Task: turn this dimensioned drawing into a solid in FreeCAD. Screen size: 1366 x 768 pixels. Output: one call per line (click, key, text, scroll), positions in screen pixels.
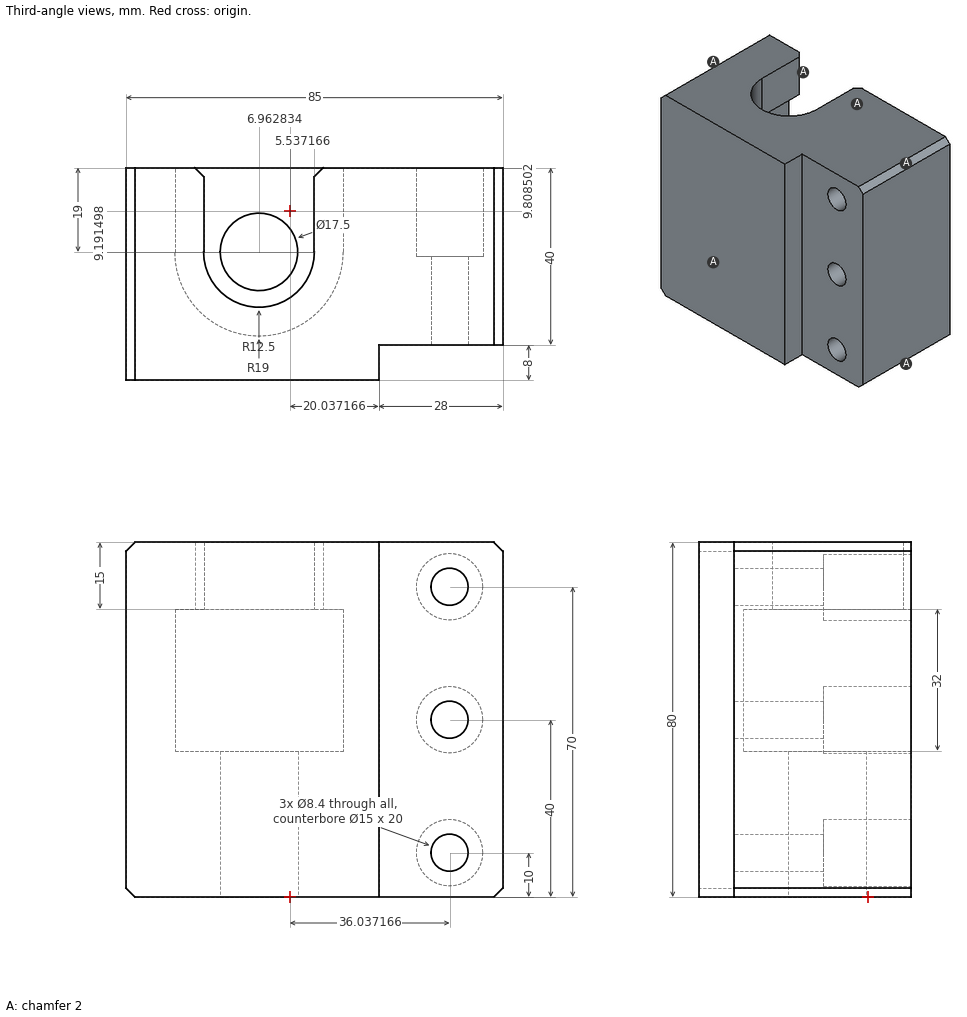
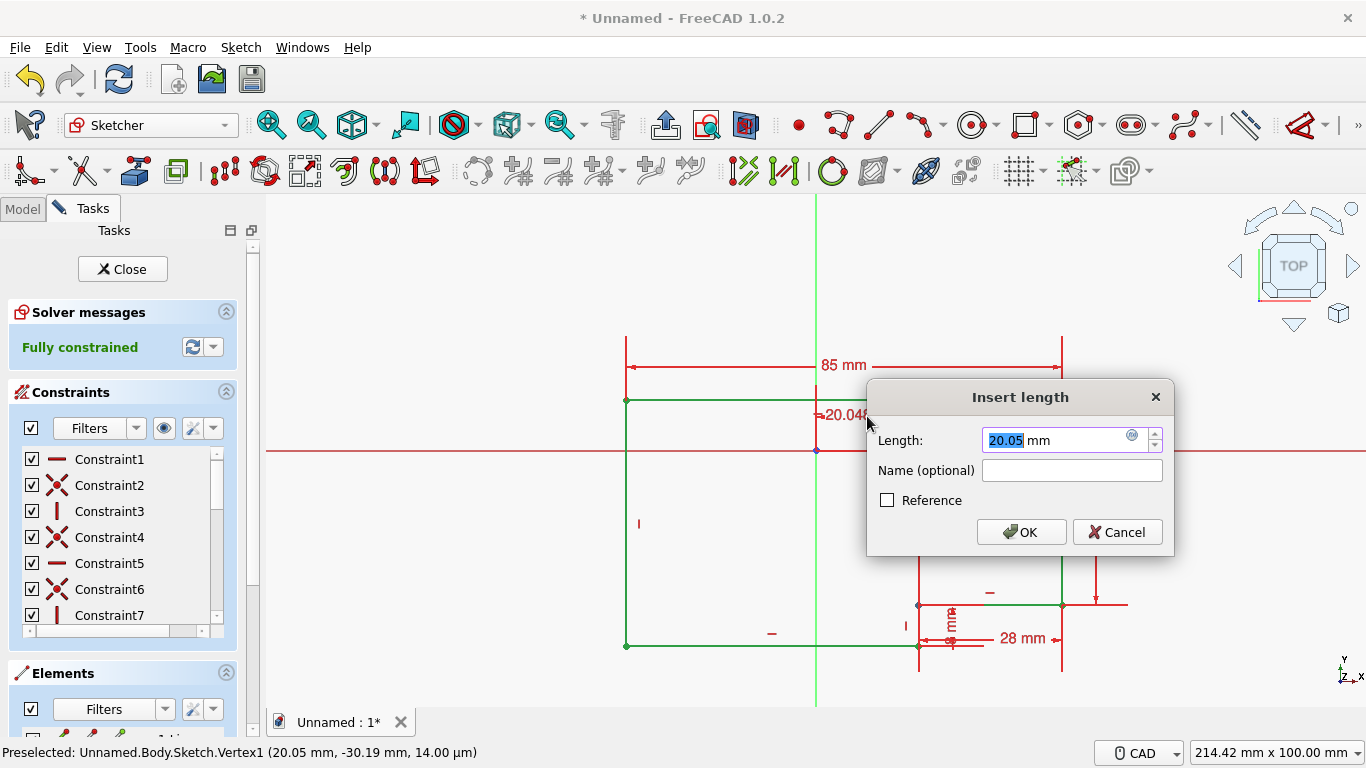
text(20.037166)
key(Return)
key(Escape)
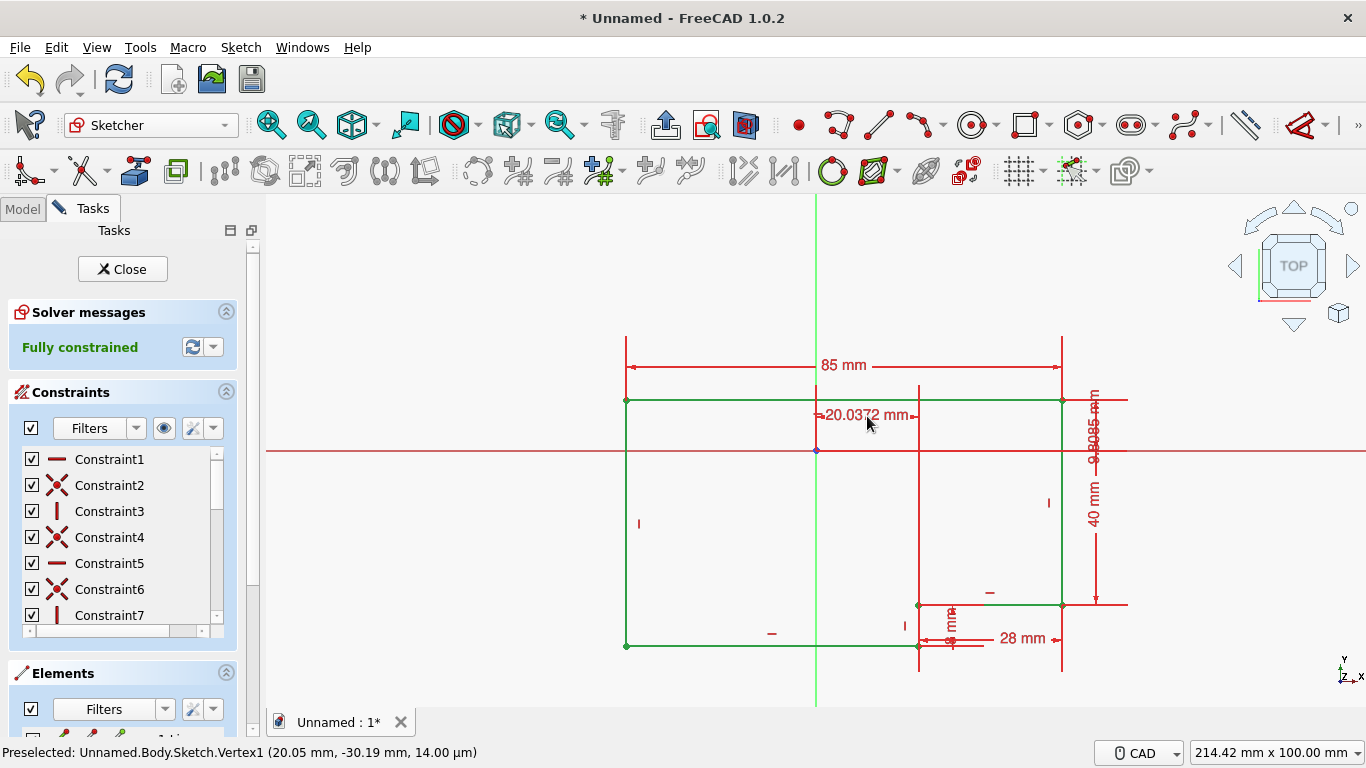
click(123, 269)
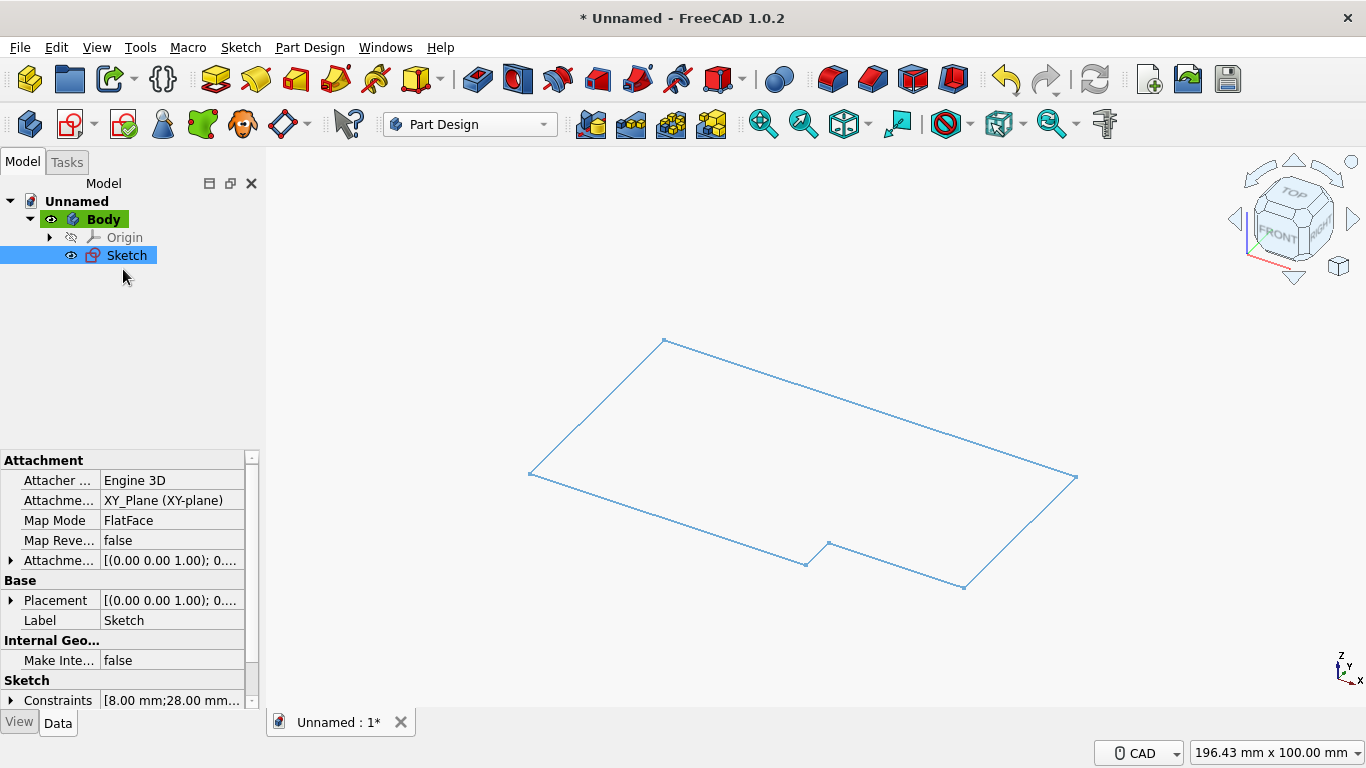
click(216, 80)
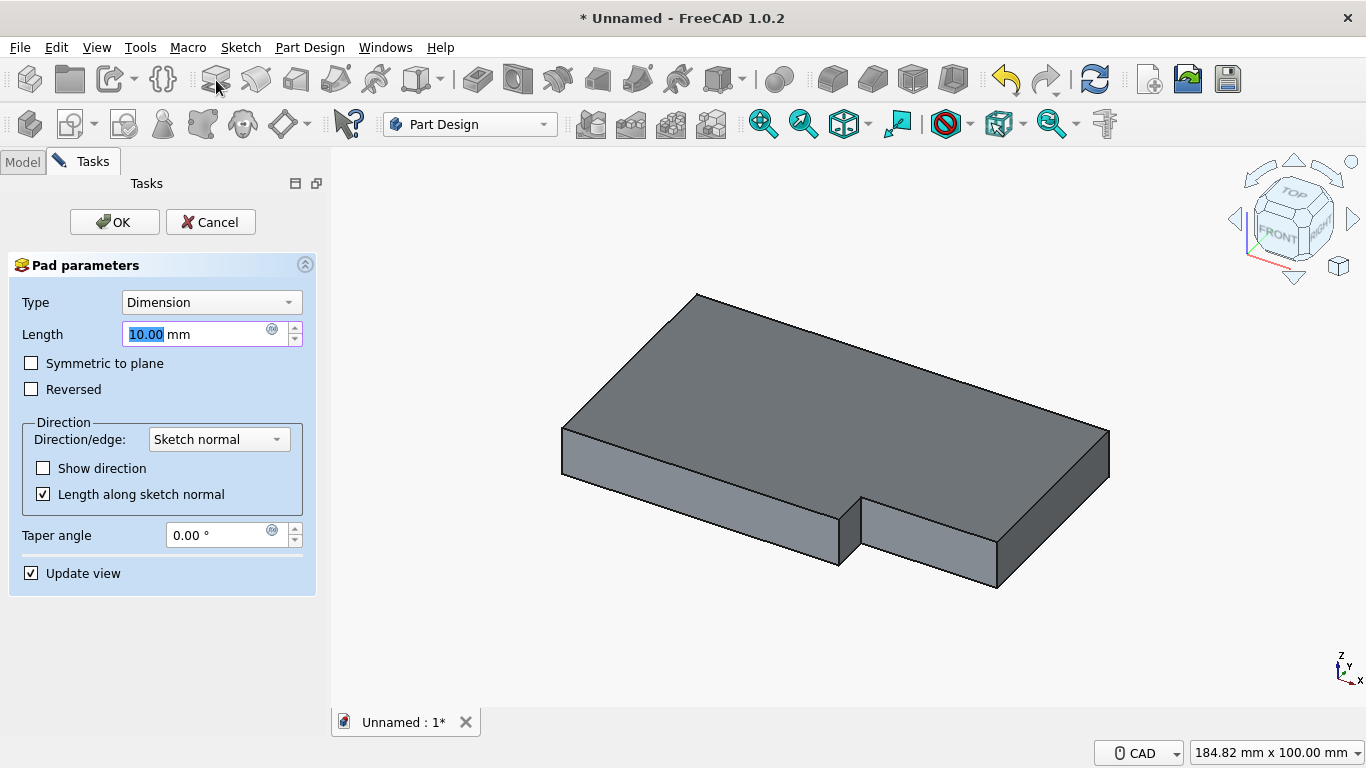
text(80)
key(Tab)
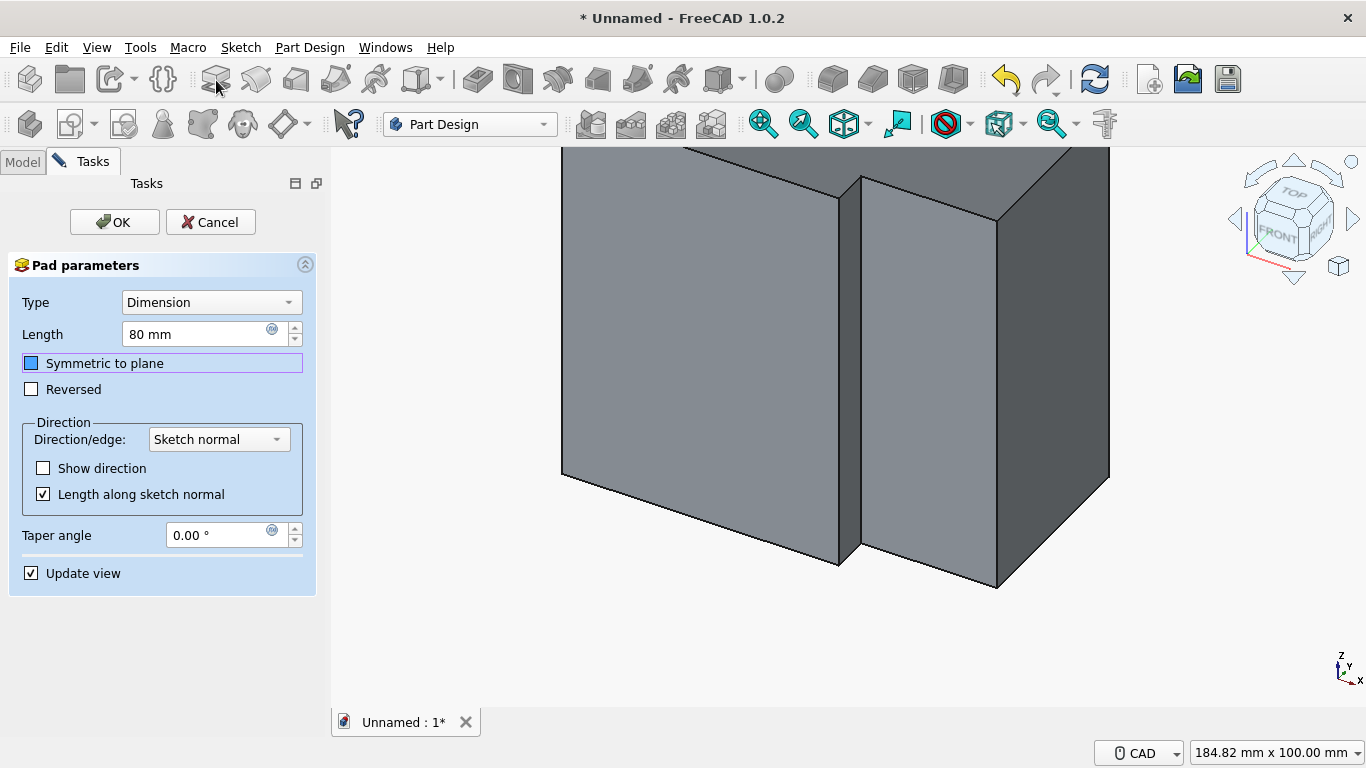
click(115, 222)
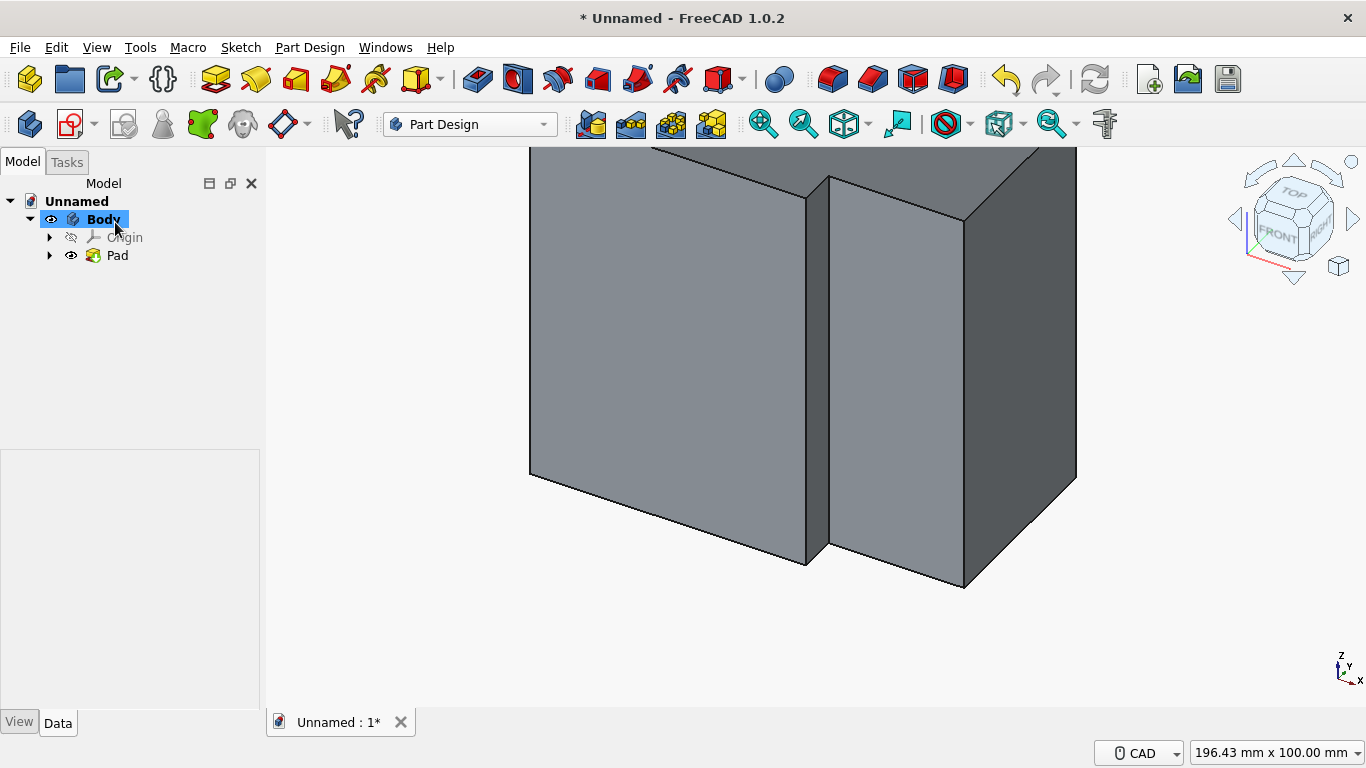
click(764, 124)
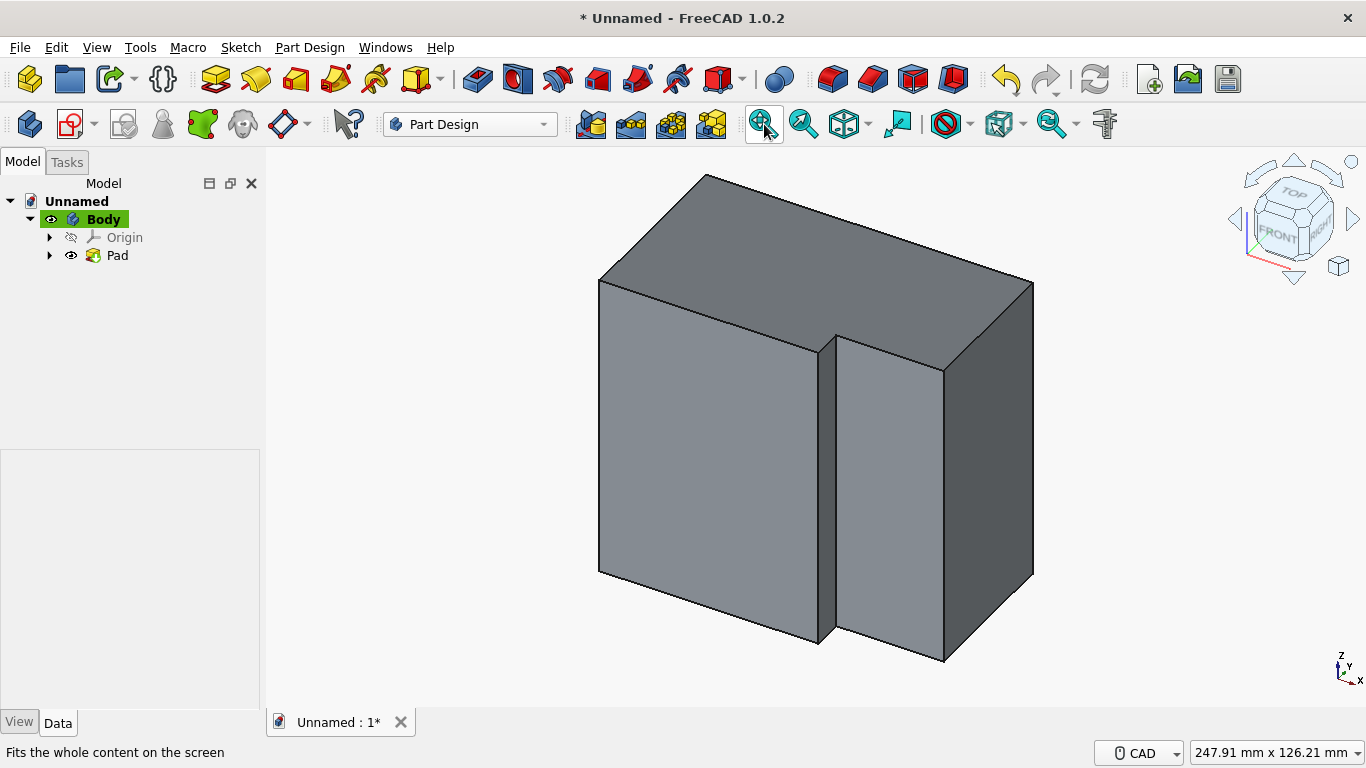
click(769, 265)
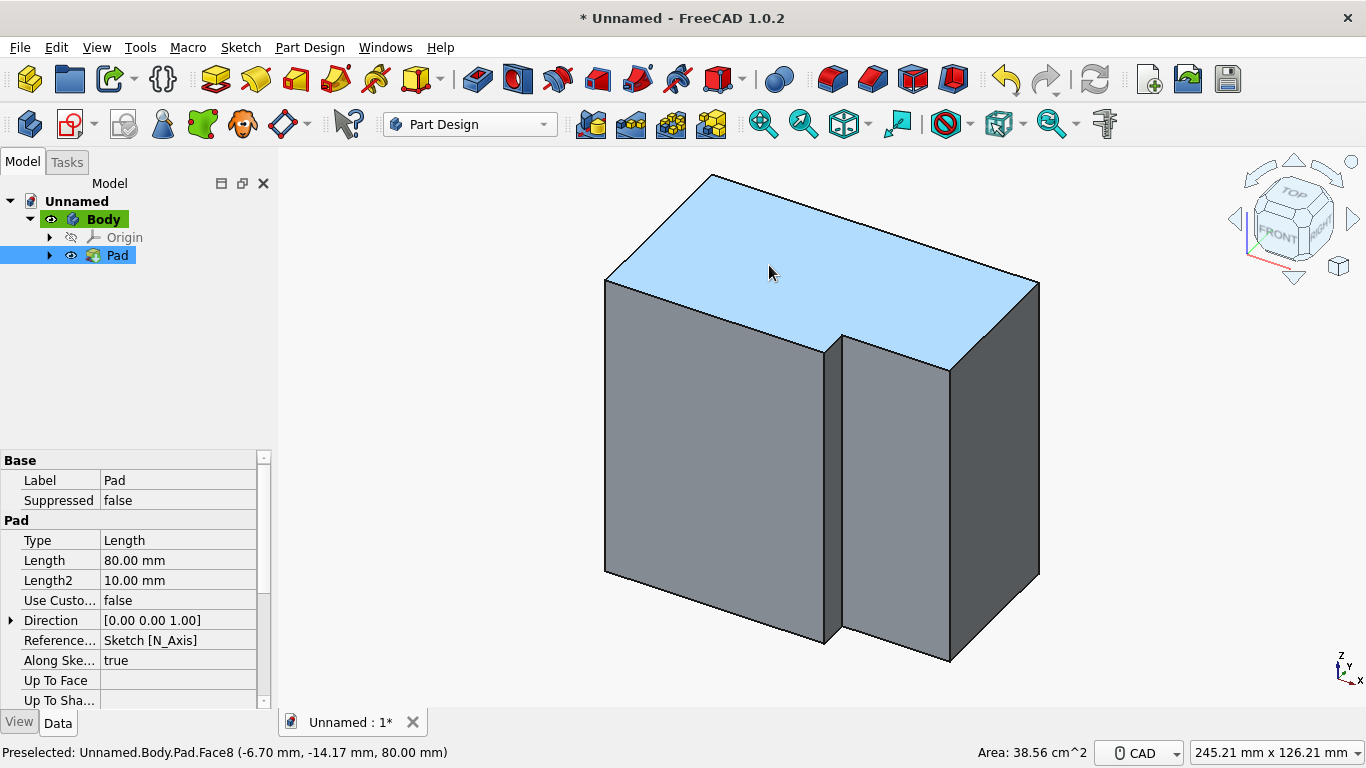
click(70, 124)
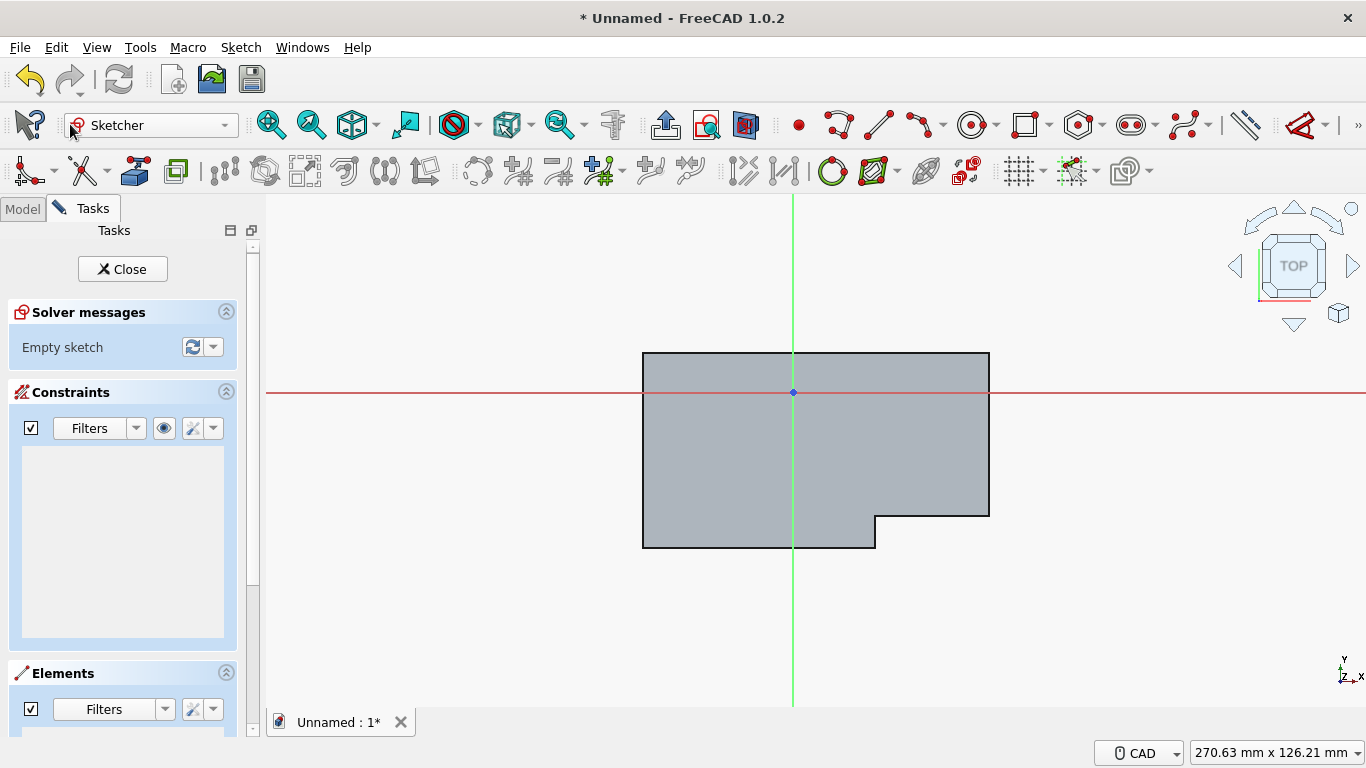
scroll(775, 397, up, 5)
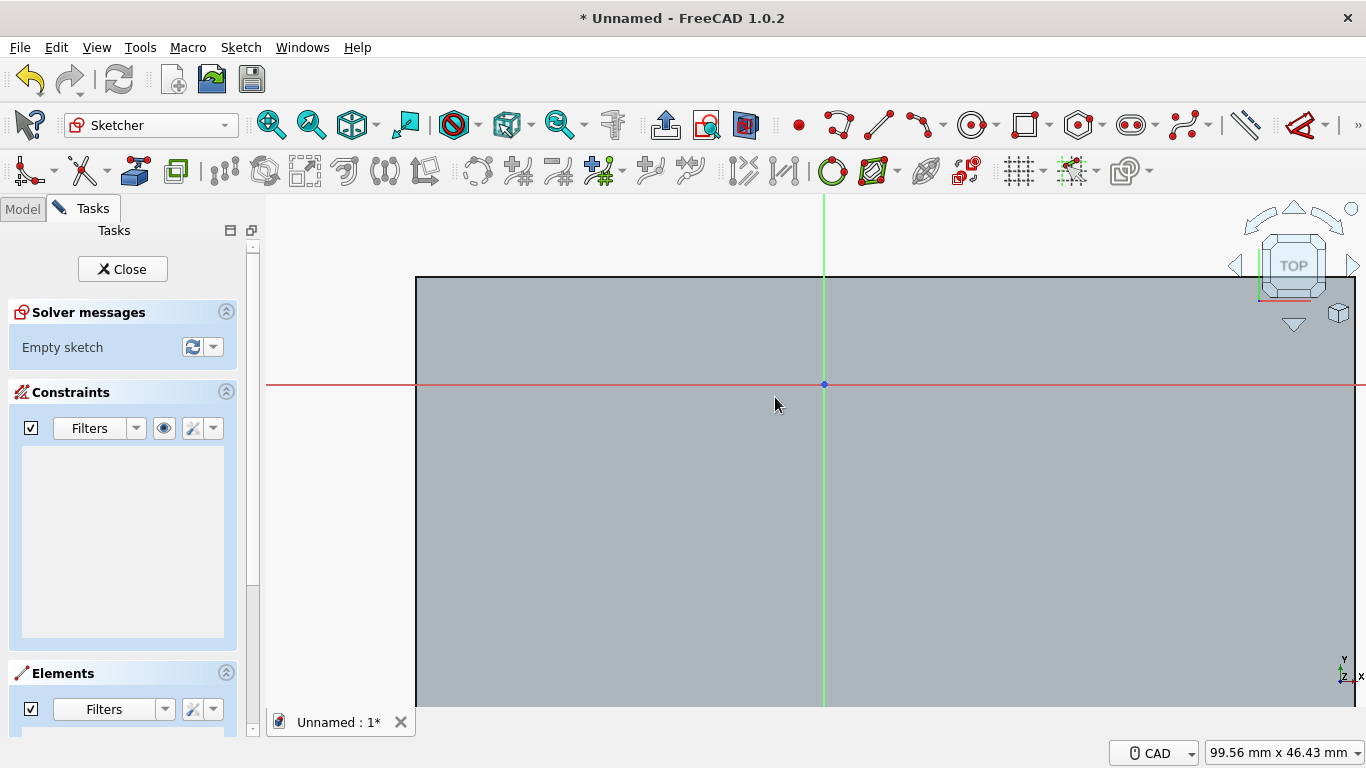
click(840, 126)